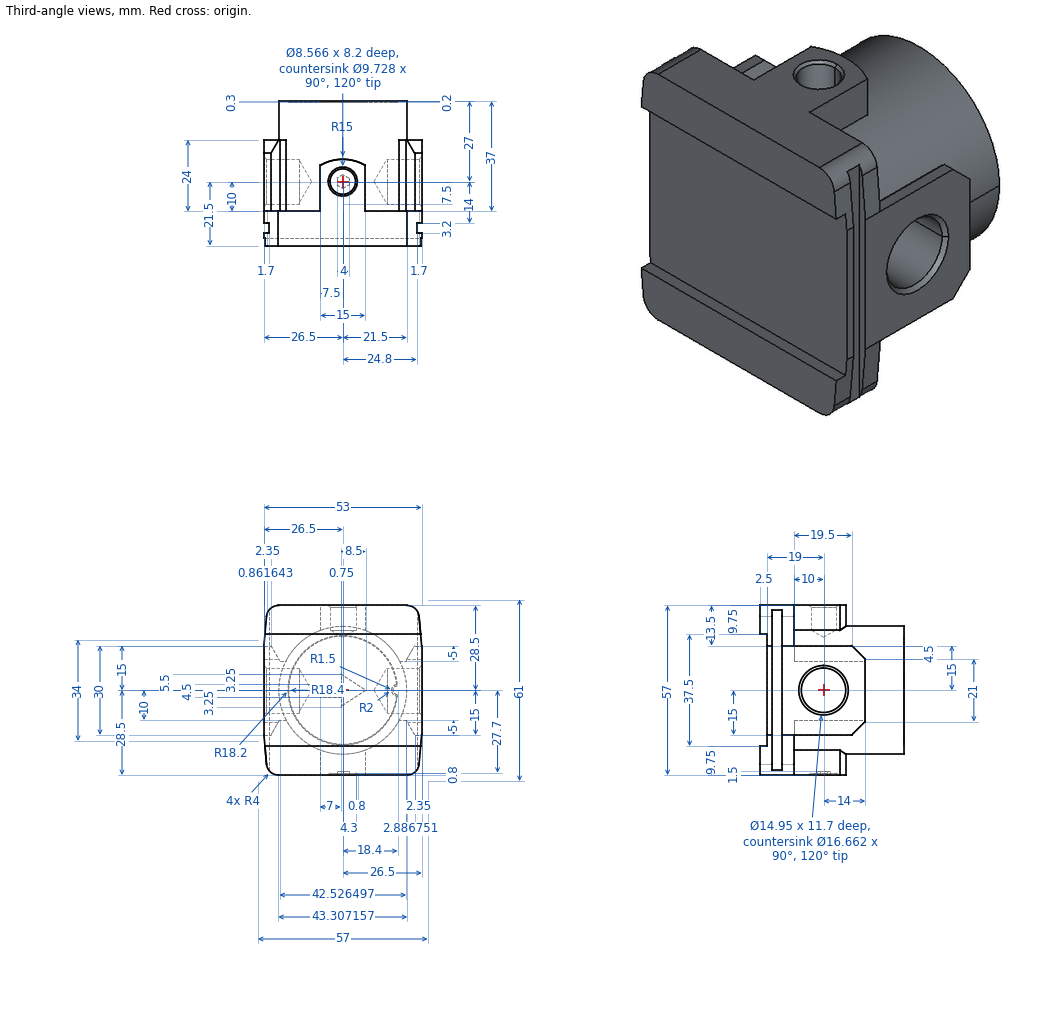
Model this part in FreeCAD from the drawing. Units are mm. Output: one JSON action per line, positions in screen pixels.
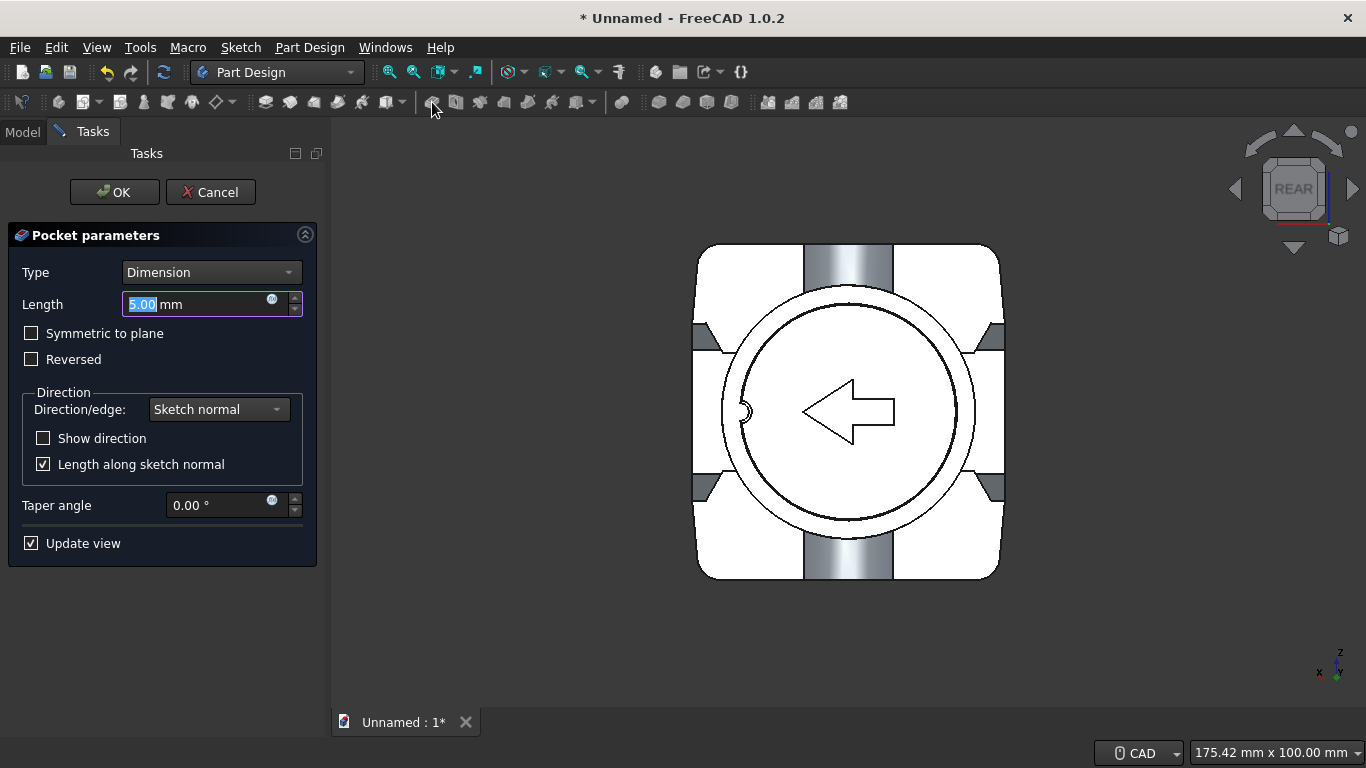
{"action": "type", "text": "0.2"}
{"action": "key", "text": "Tab"}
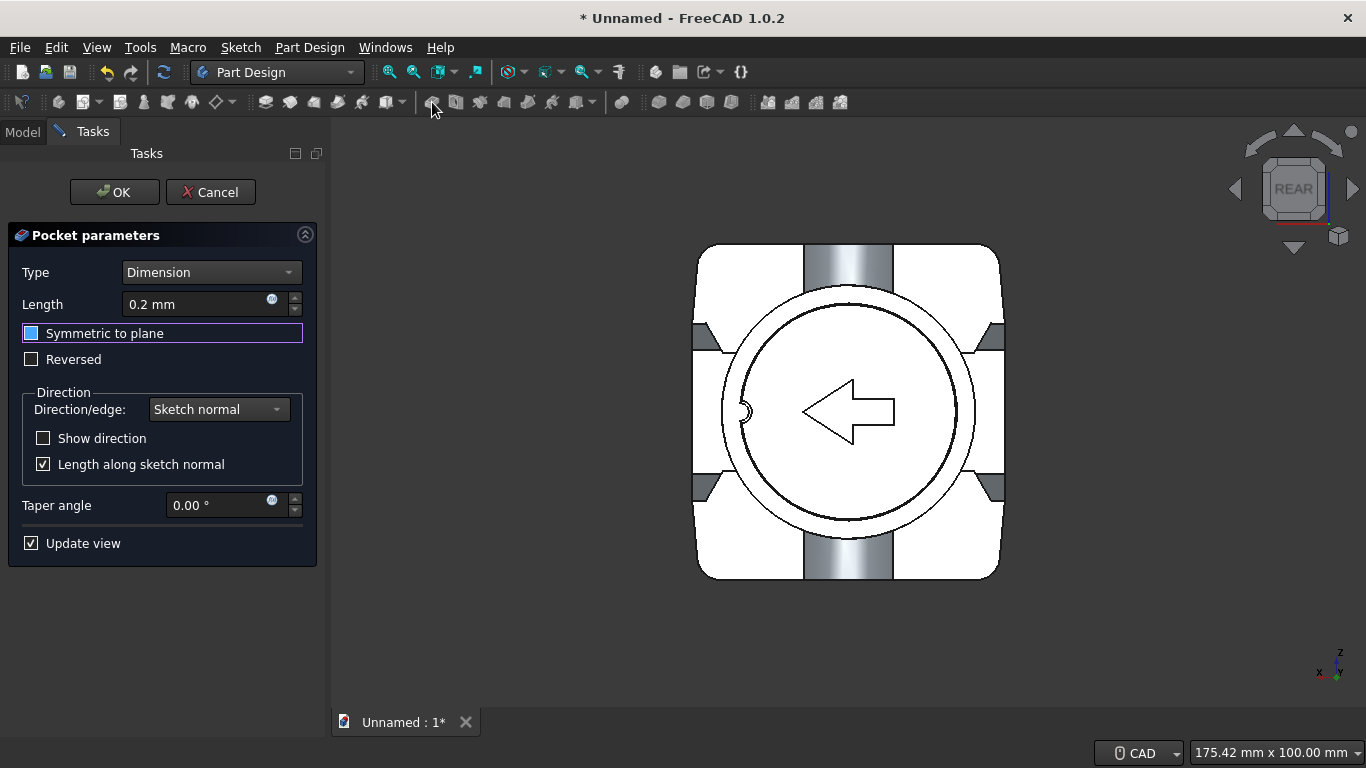
{"action": "left_click", "coordinate": [115, 192]}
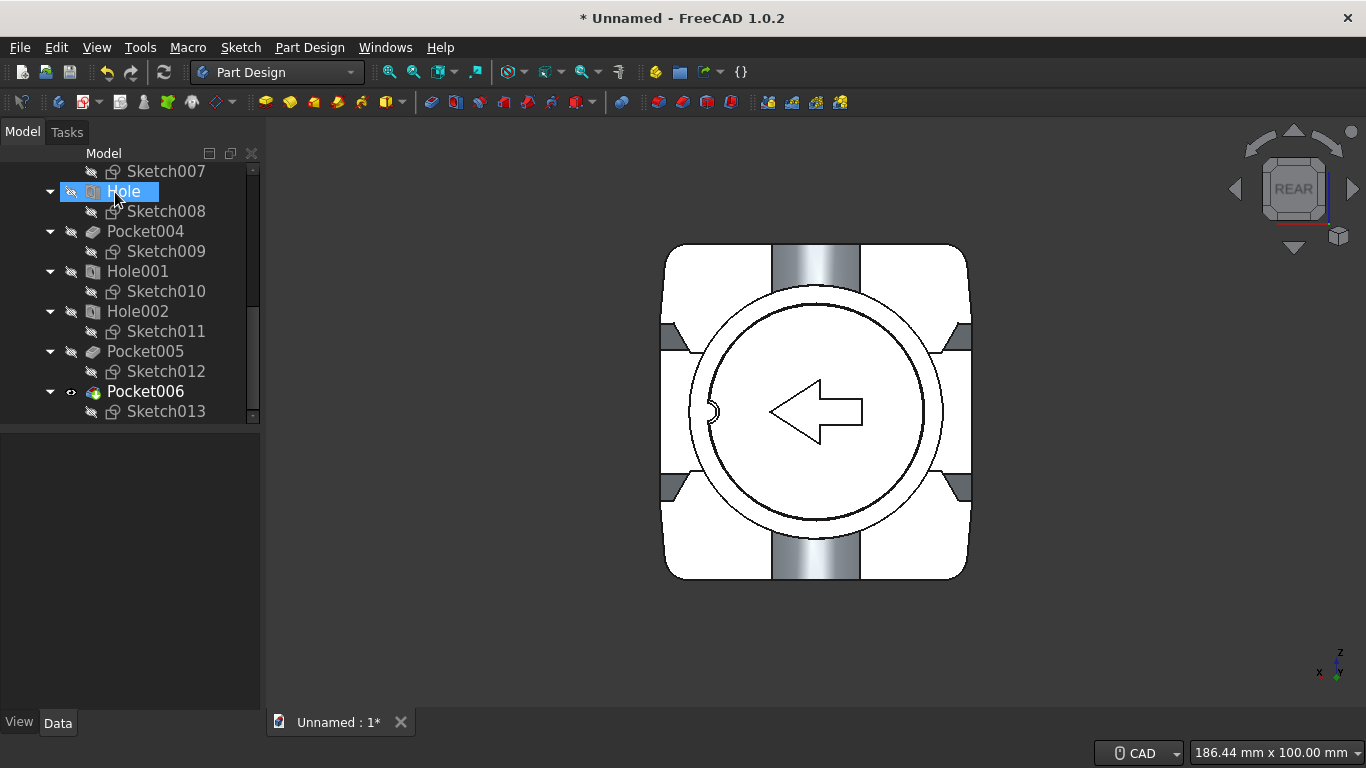
{"action": "key", "text": "0"}